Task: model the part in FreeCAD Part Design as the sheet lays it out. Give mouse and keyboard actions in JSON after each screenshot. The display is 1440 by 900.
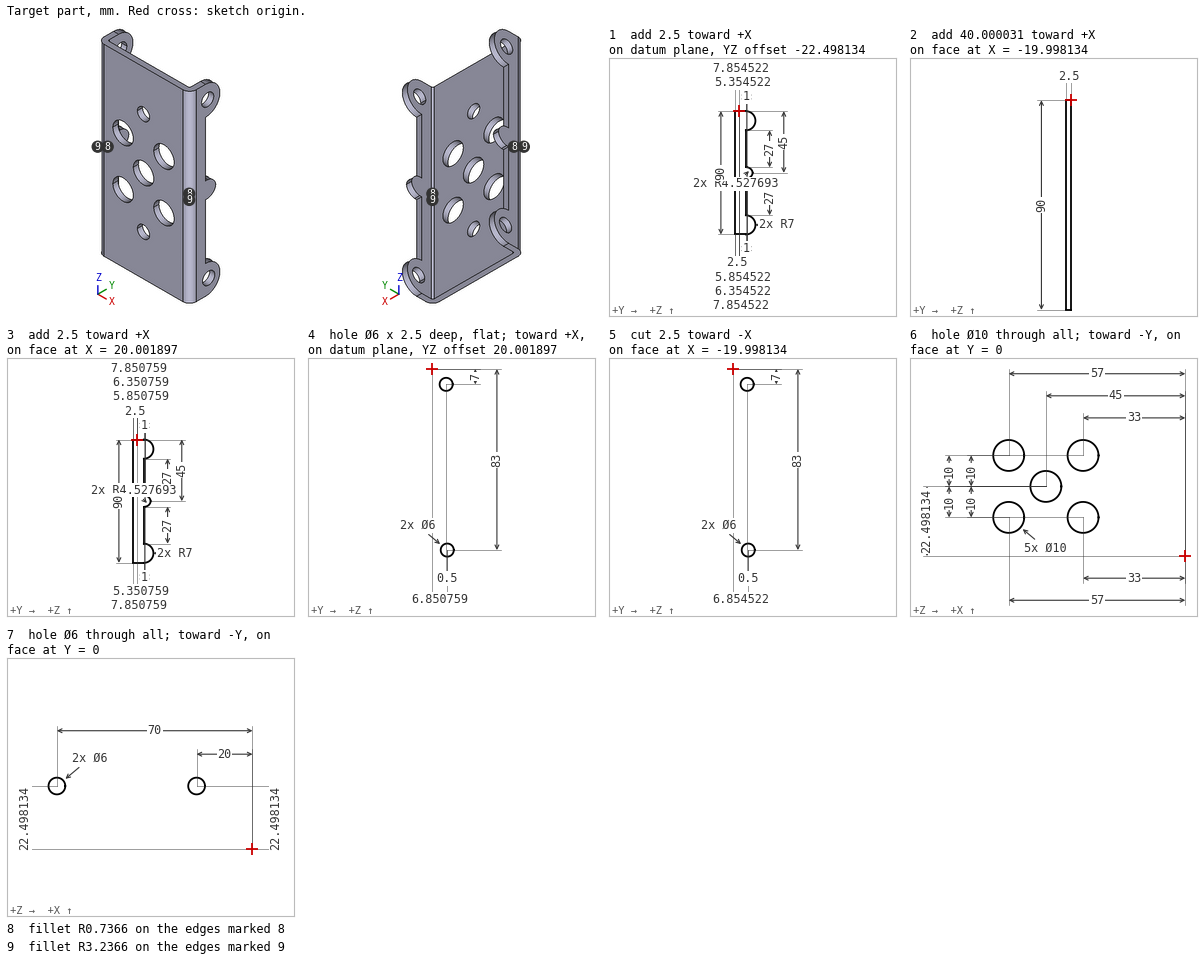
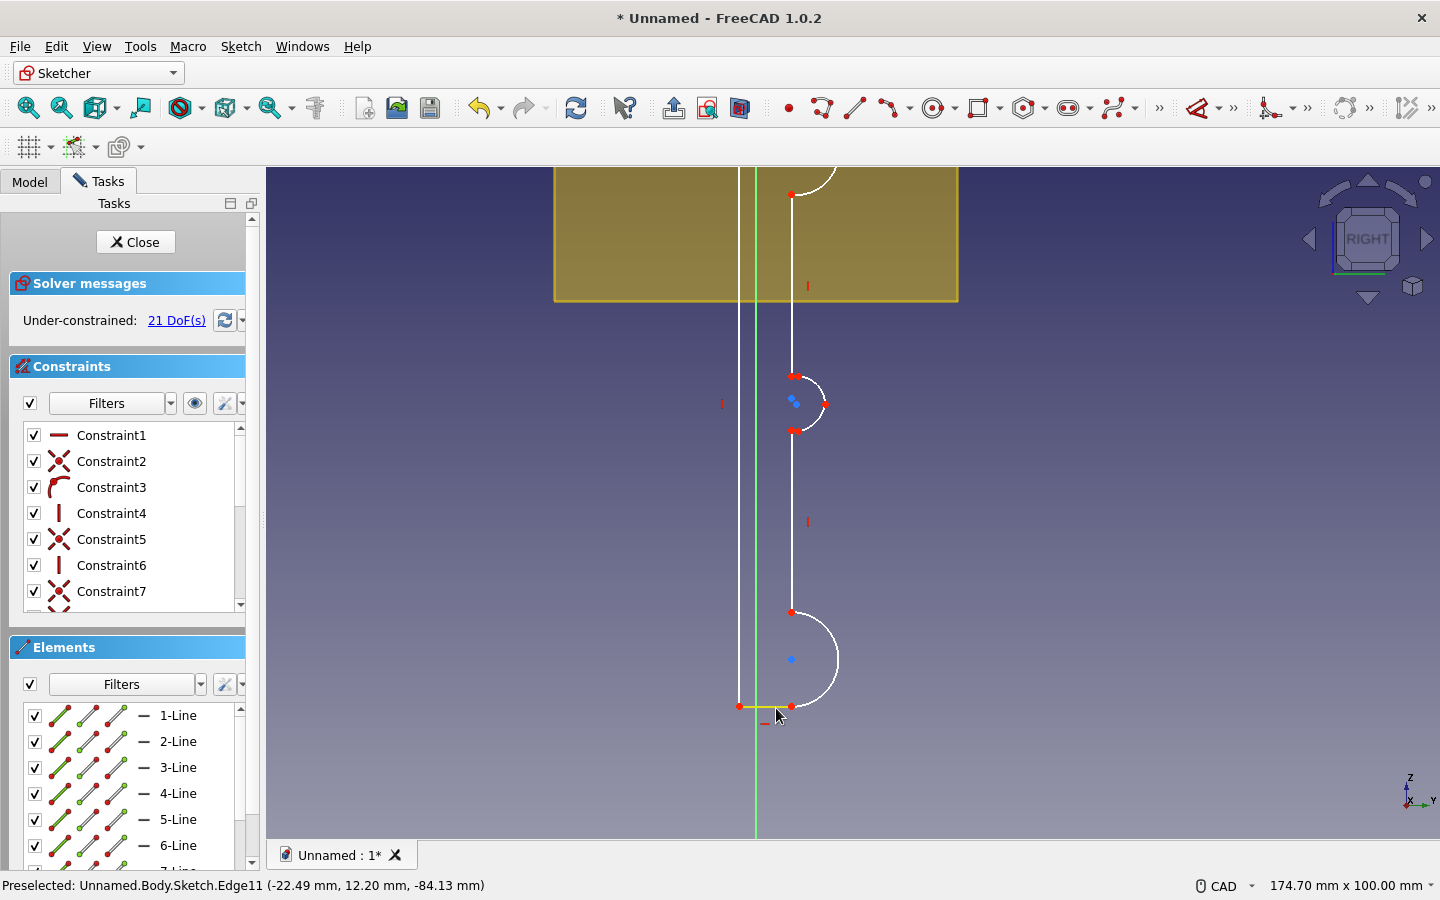
{"action": "left_click", "coordinate": [776, 707]}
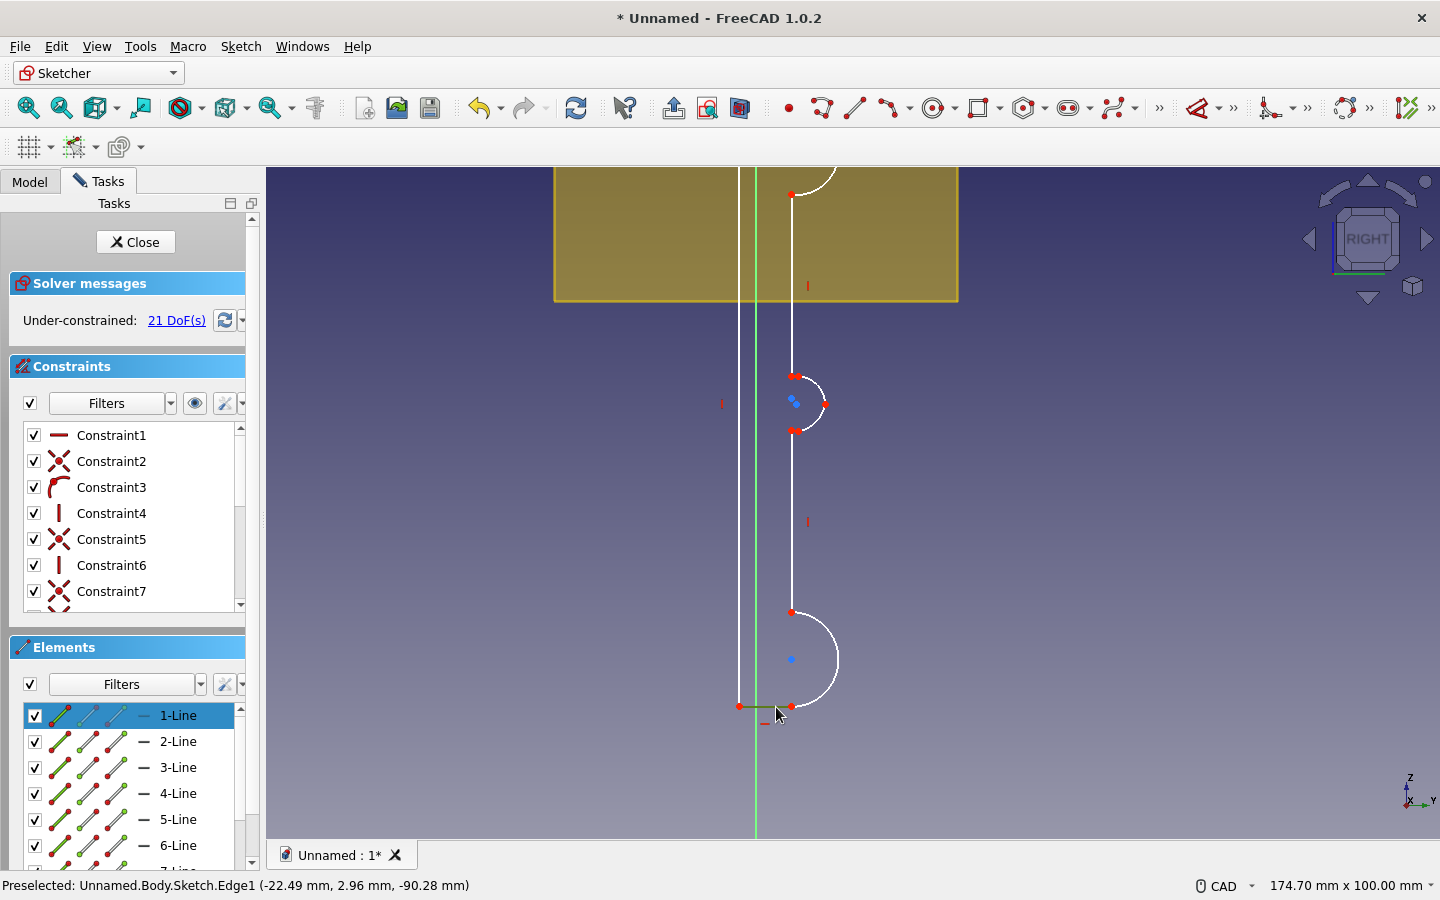
{"action": "left_click", "coordinate": [829, 687]}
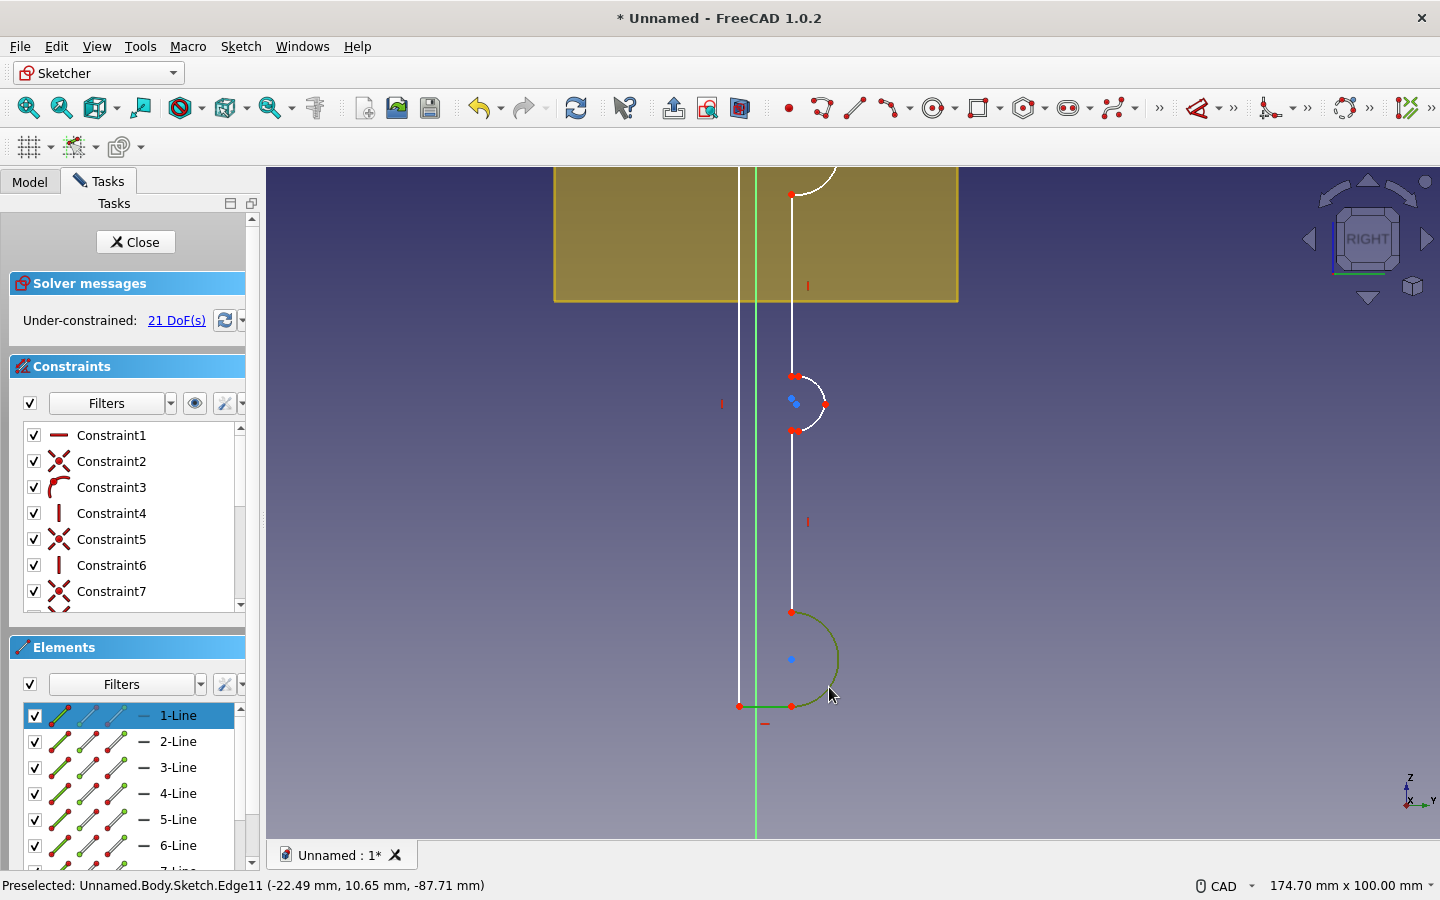
{"action": "key", "text": "t"}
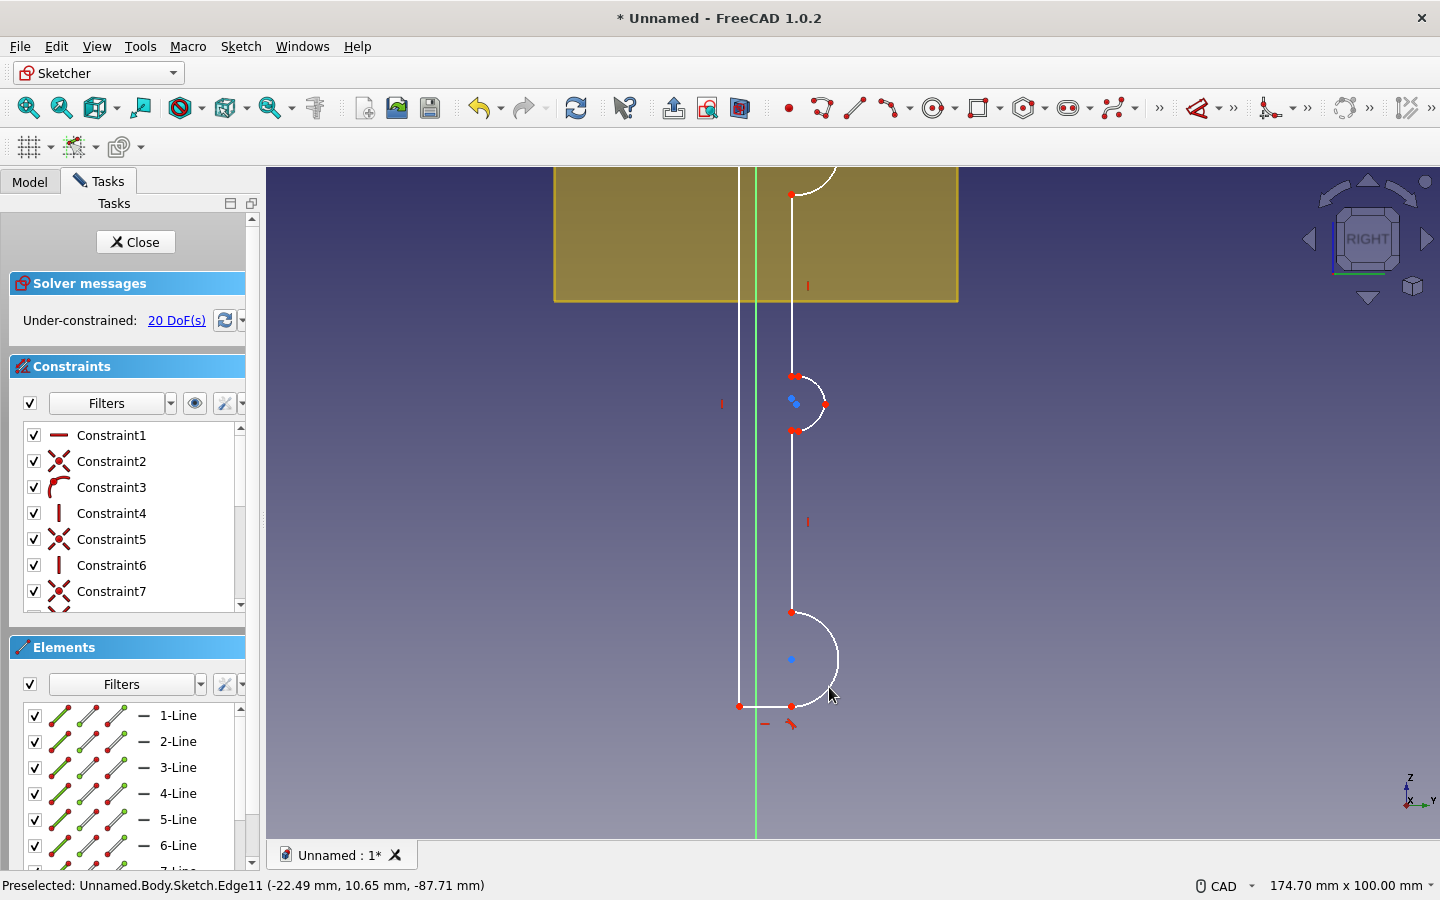
{"action": "scroll", "coordinate": [775, 707], "scroll_direction": "down", "scroll_amount": 2}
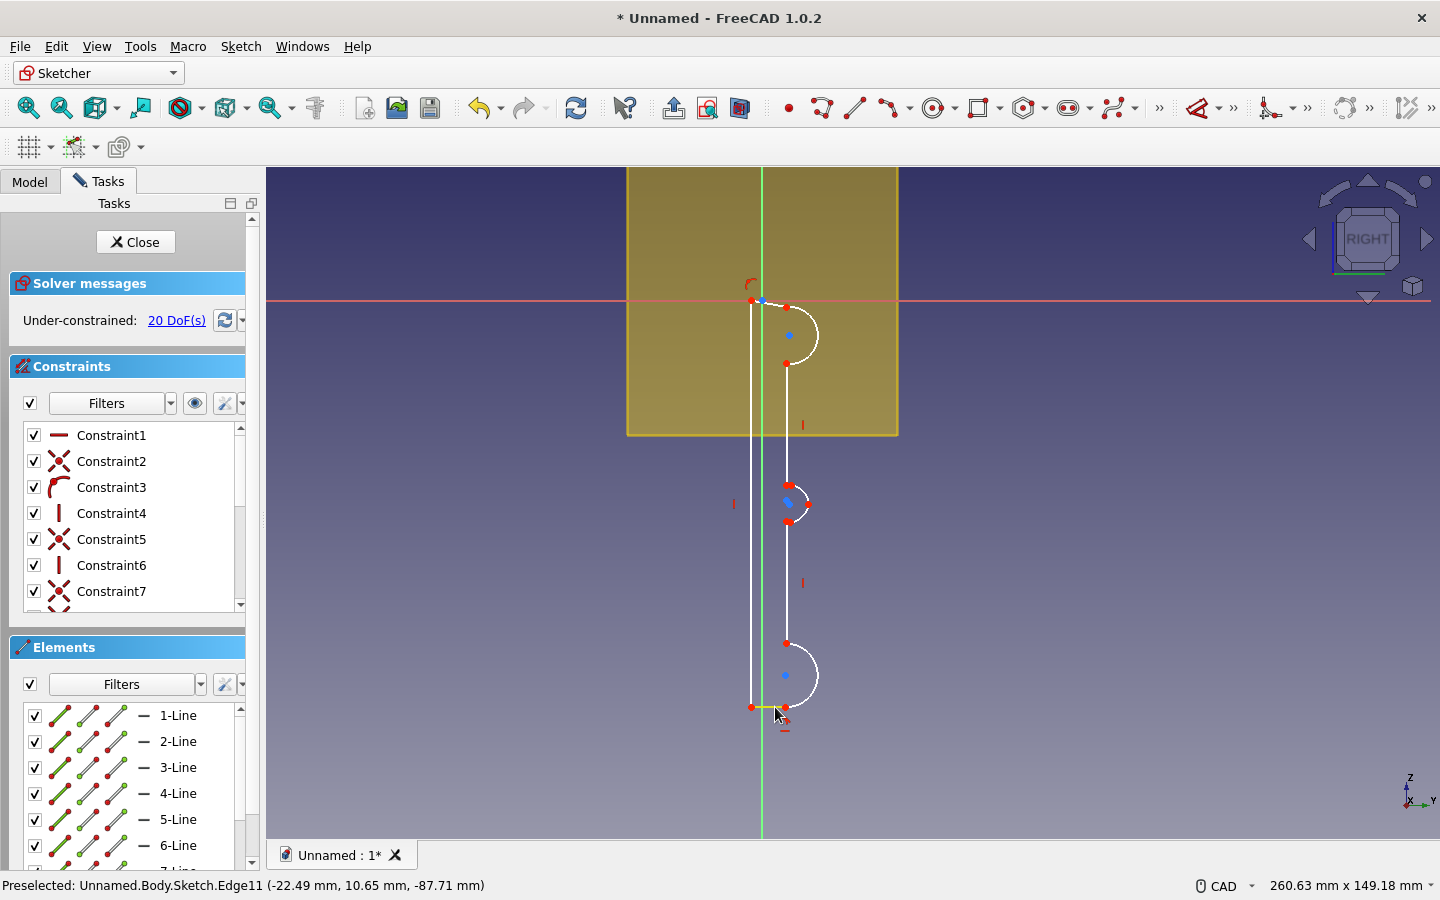
{"action": "scroll", "coordinate": [762, 302], "scroll_direction": "up", "scroll_amount": 2}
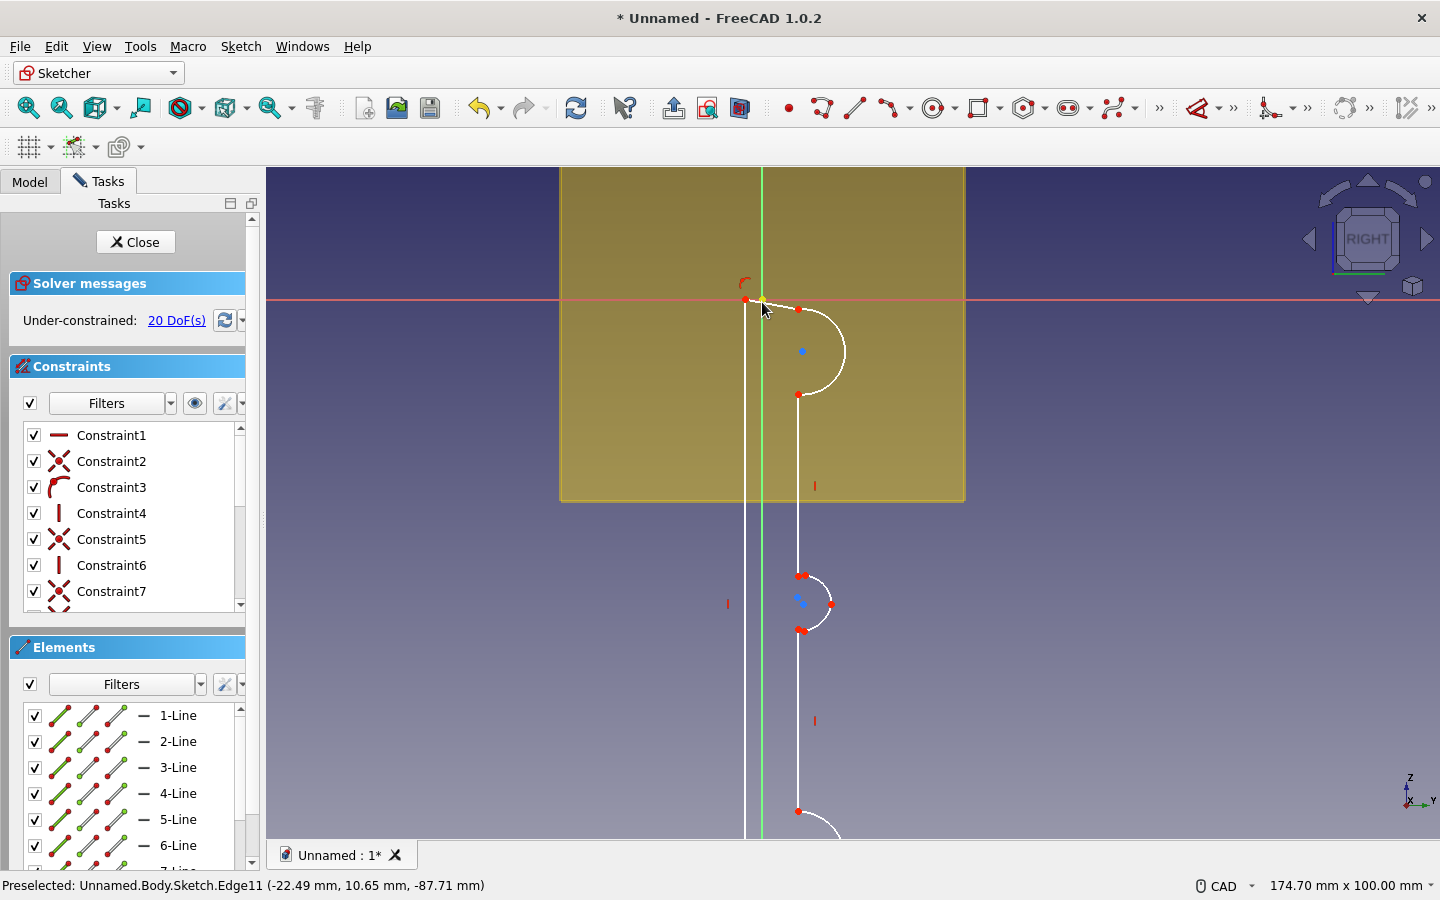
{"action": "left_click", "coordinate": [788, 307]}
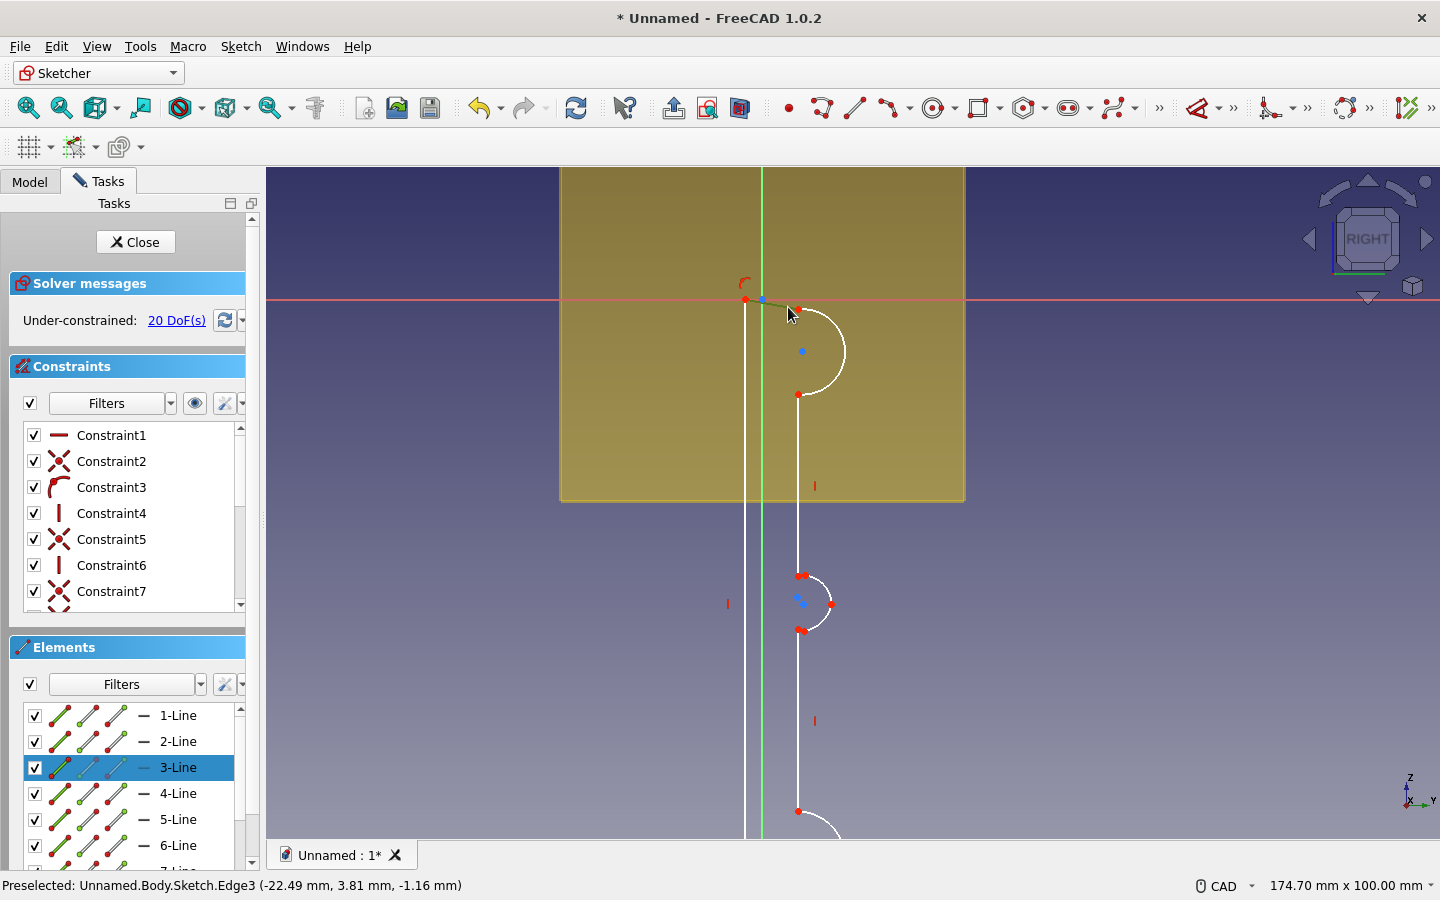
{"action": "left_click", "coordinate": [836, 378]}